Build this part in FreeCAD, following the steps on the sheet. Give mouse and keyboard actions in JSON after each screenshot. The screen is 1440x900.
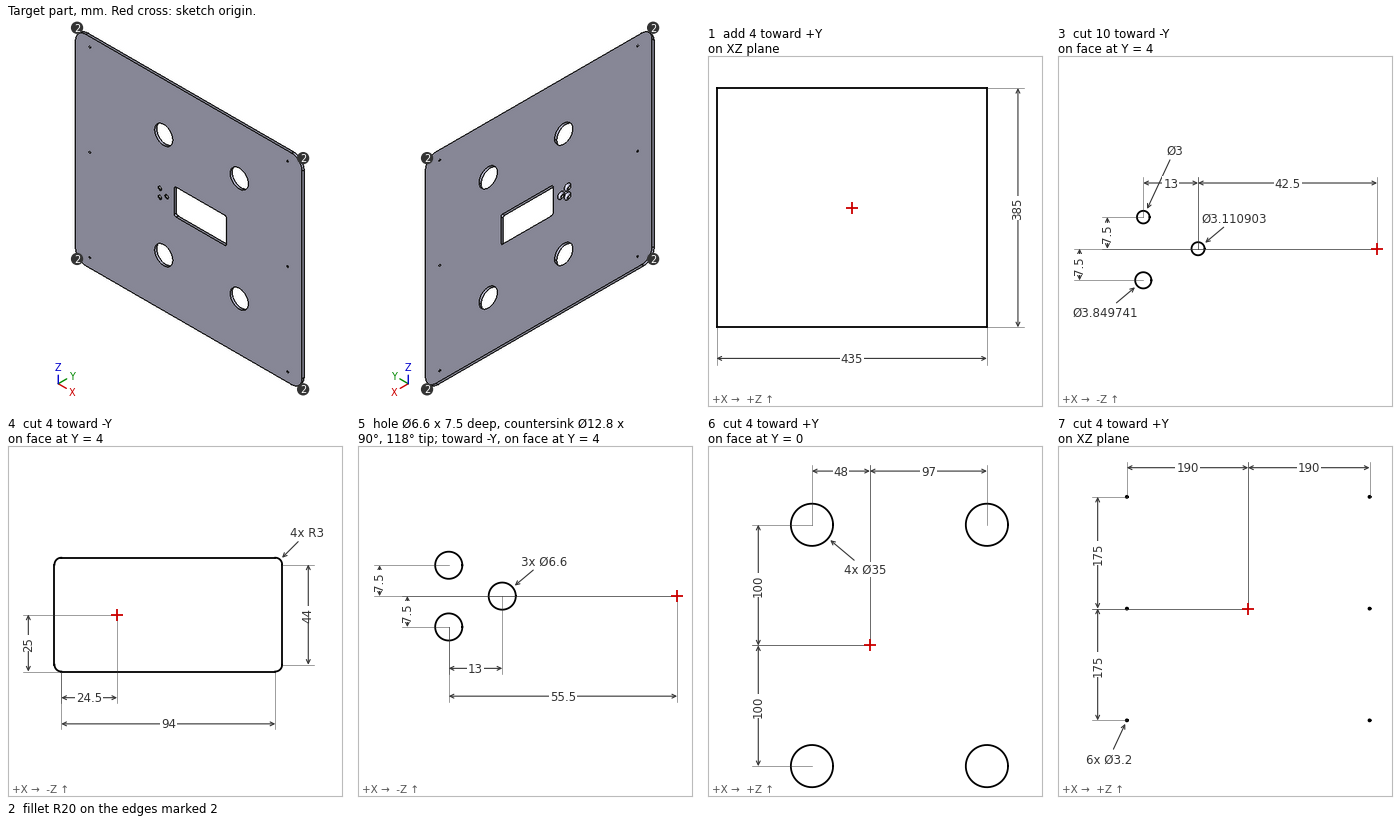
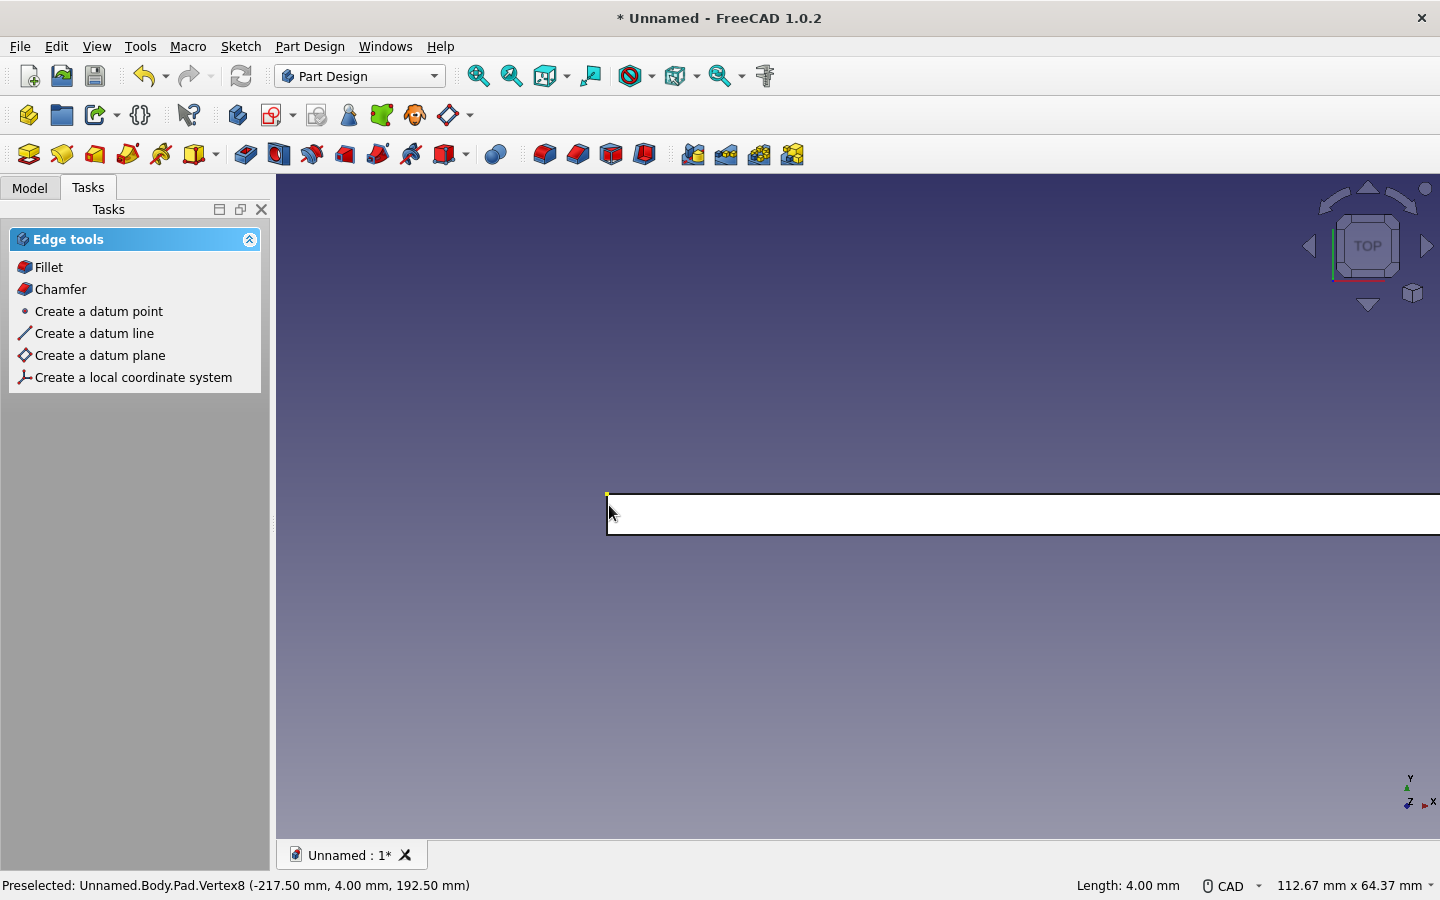
{"action": "left_click", "coordinate": [607, 514], "text": "ctrl"}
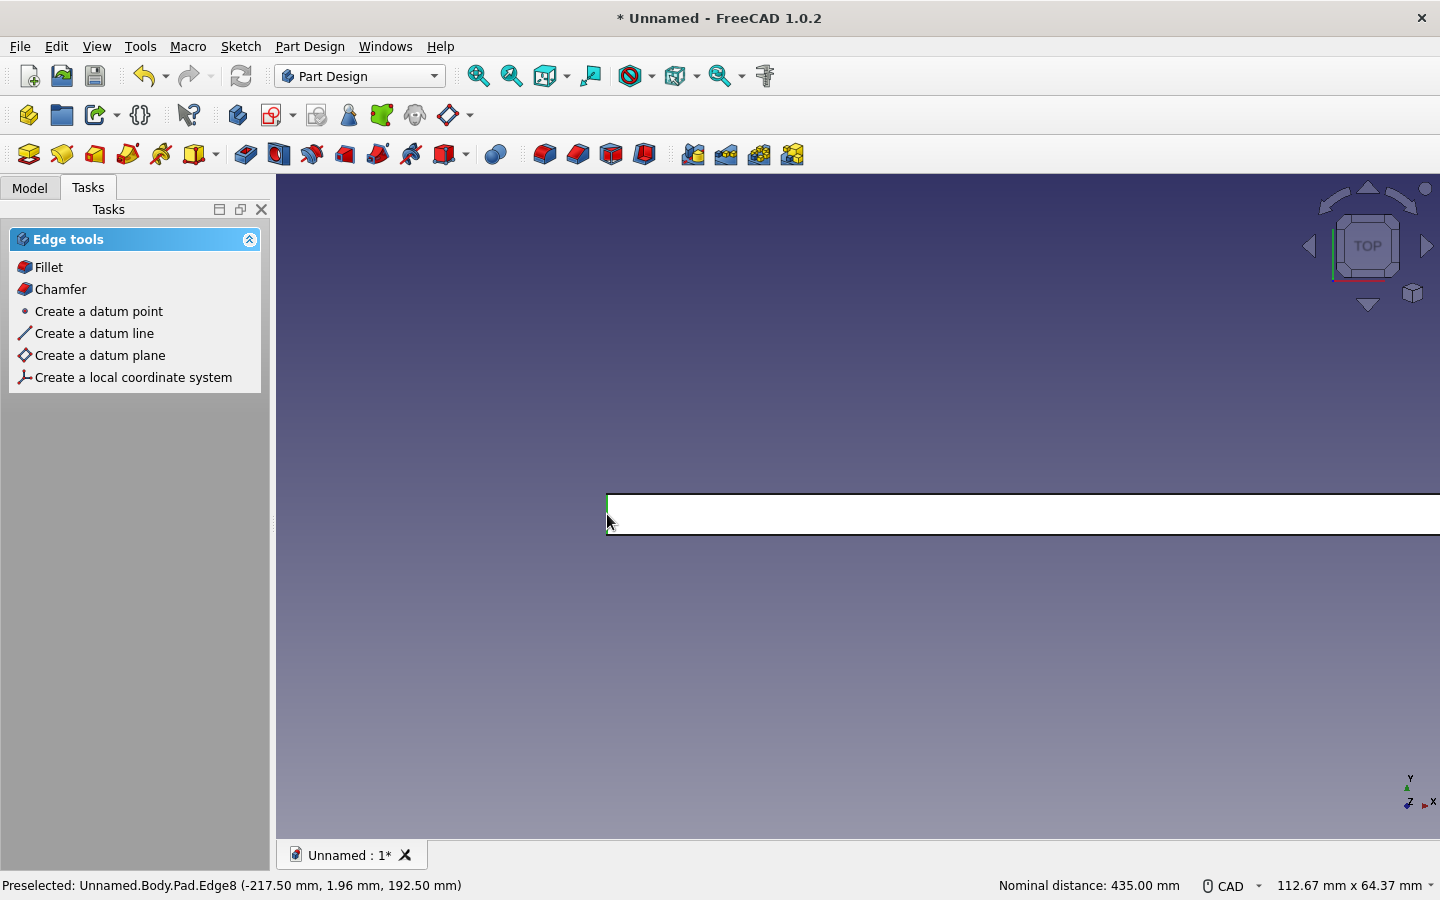
{"action": "left_click", "coordinate": [479, 76]}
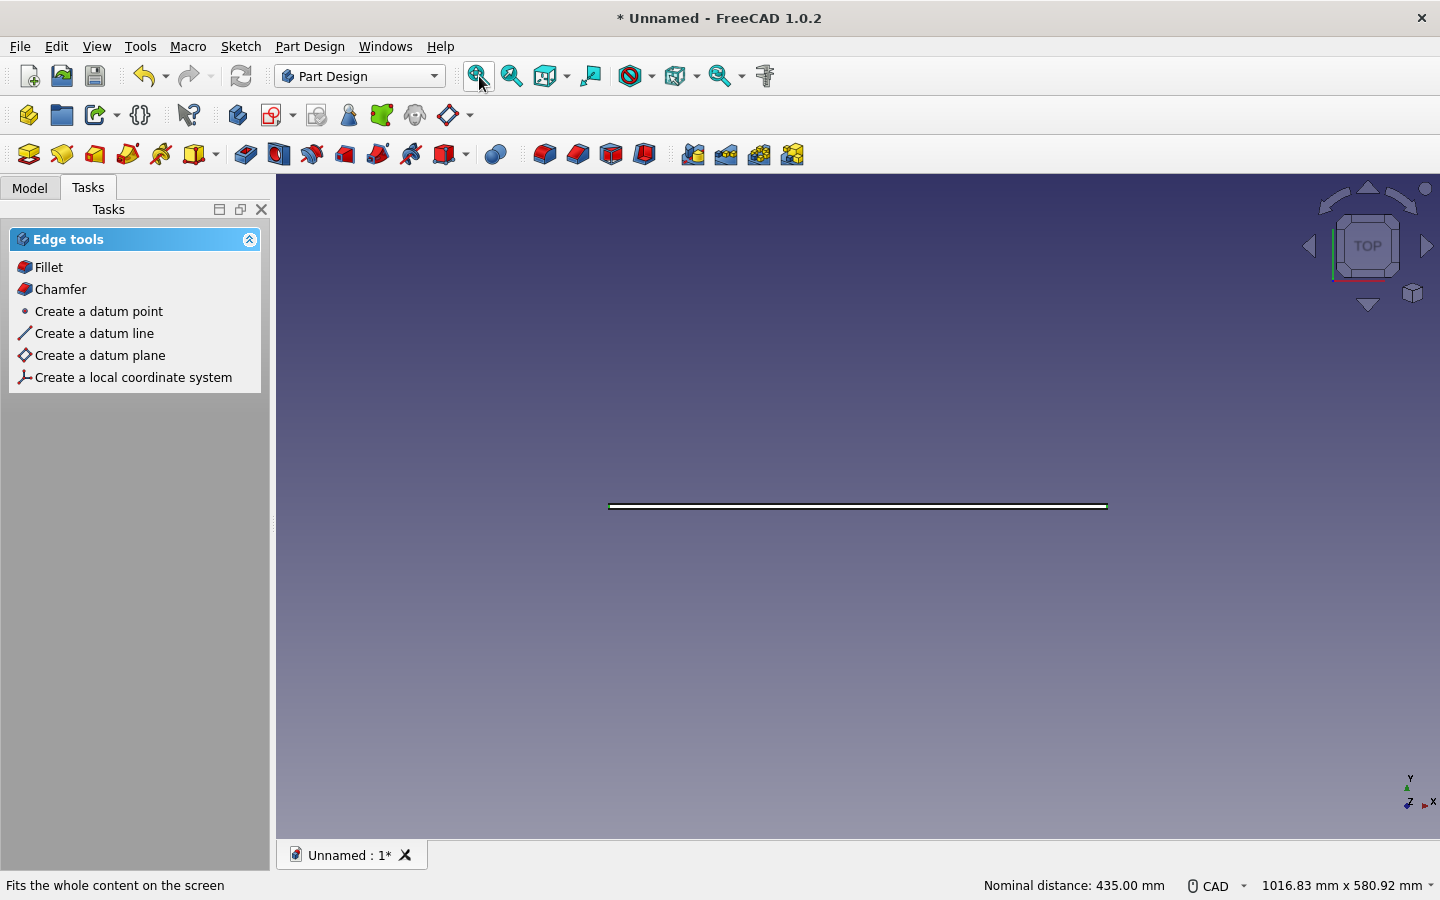
{"action": "key", "text": "1"}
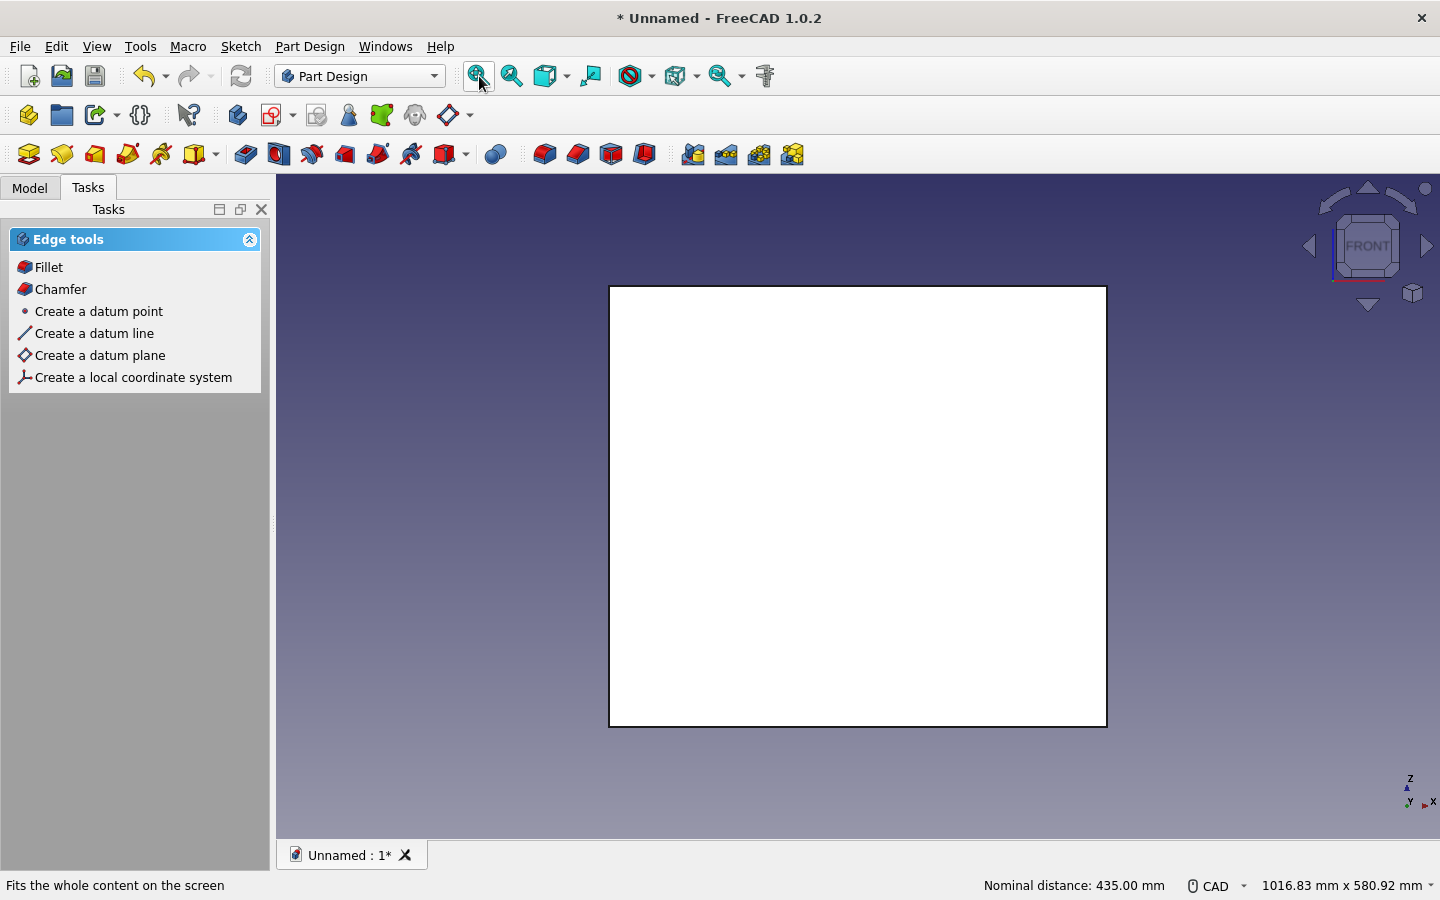
{"action": "scroll", "coordinate": [609, 726], "scroll_direction": "up", "scroll_amount": 11}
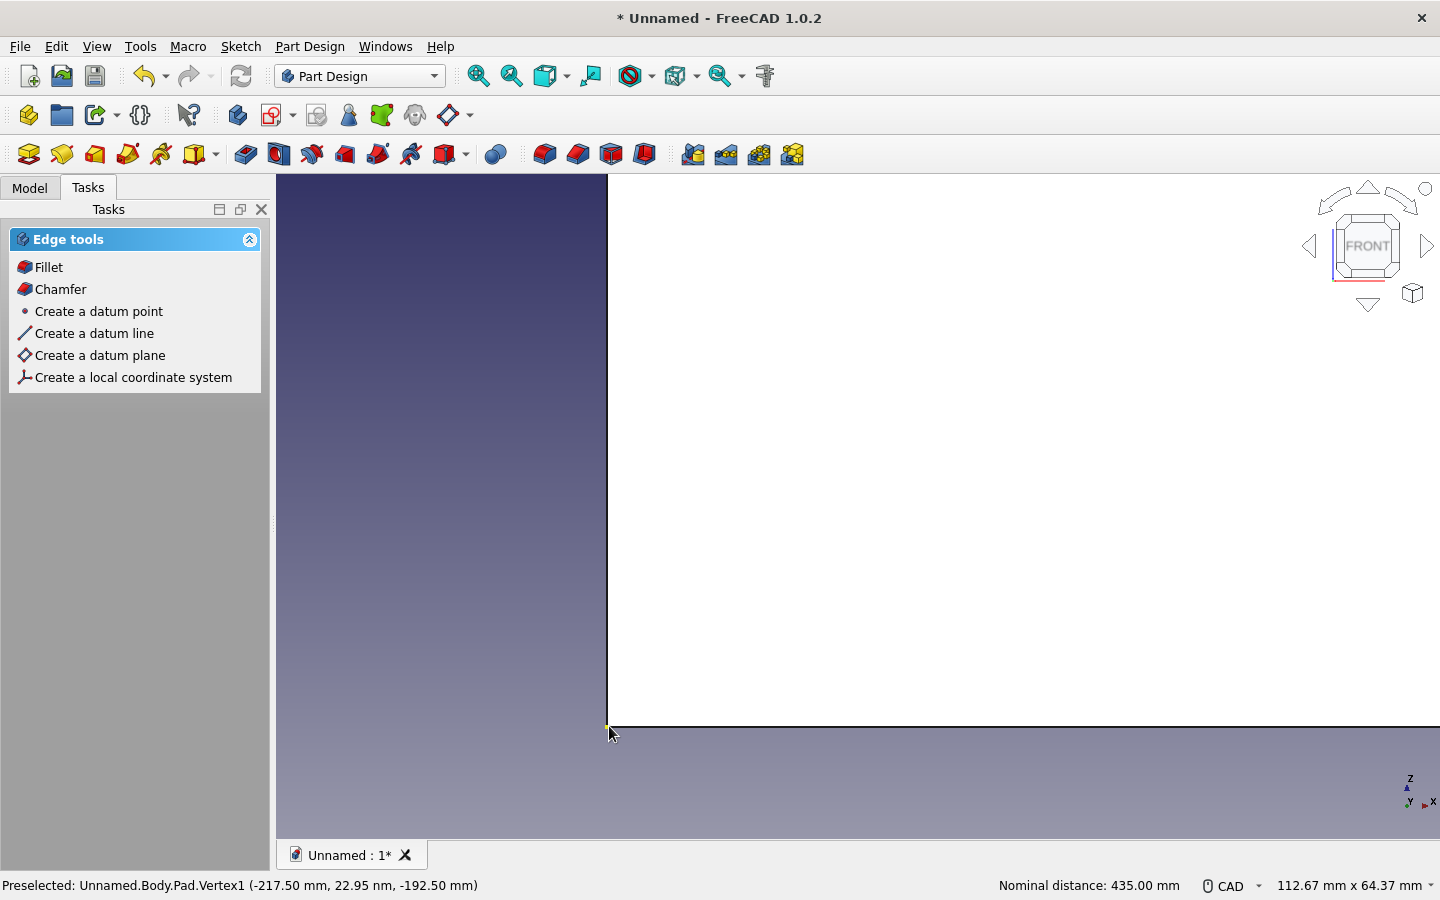
{"action": "left_click", "coordinate": [479, 76]}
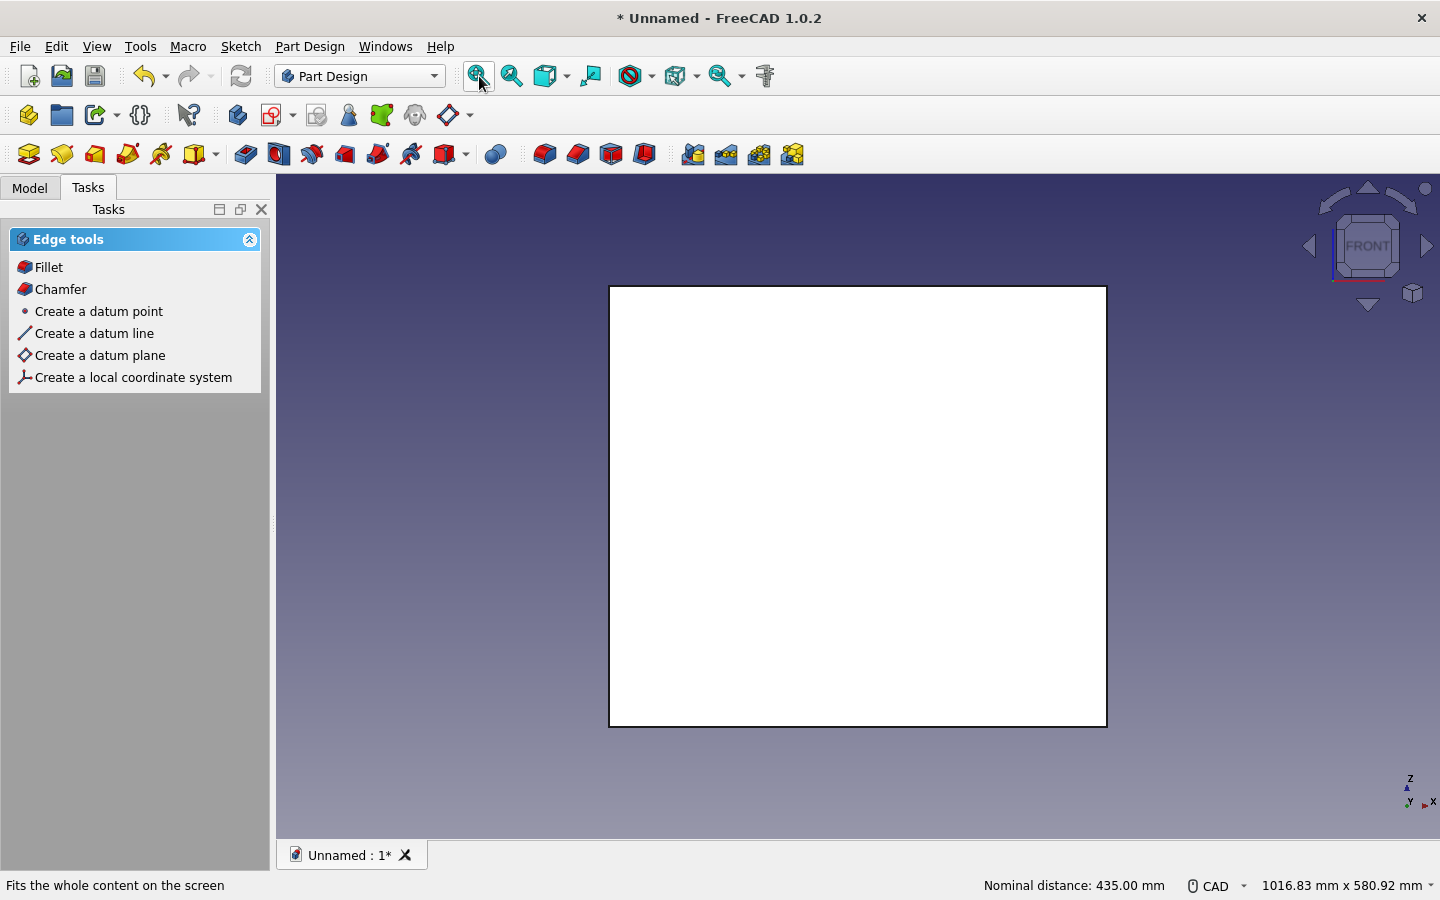
{"action": "key", "text": "3"}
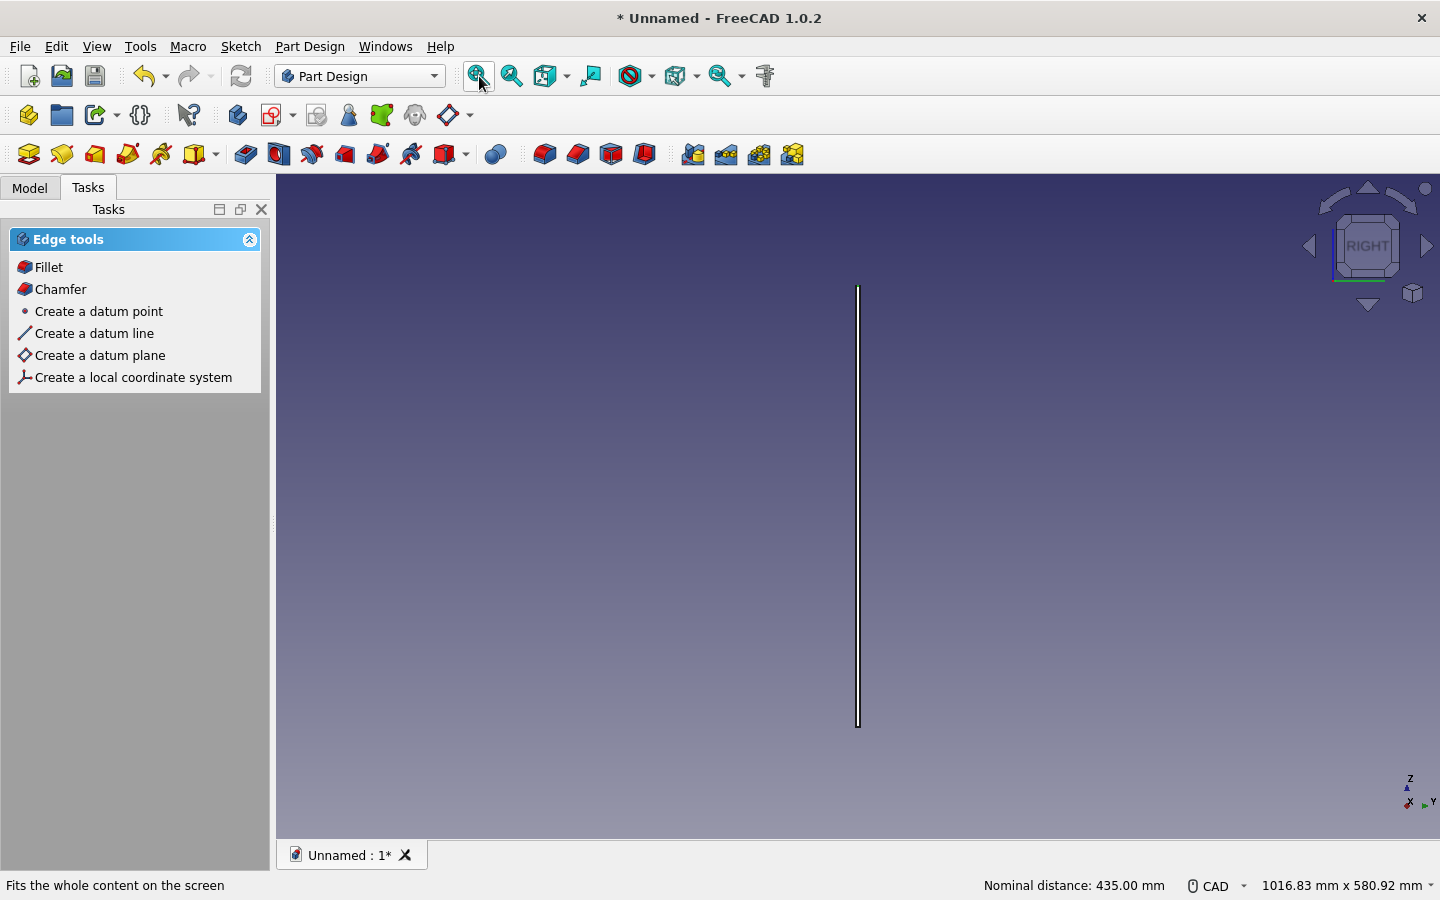
{"action": "scroll", "coordinate": [858, 726], "scroll_direction": "up", "scroll_amount": 11}